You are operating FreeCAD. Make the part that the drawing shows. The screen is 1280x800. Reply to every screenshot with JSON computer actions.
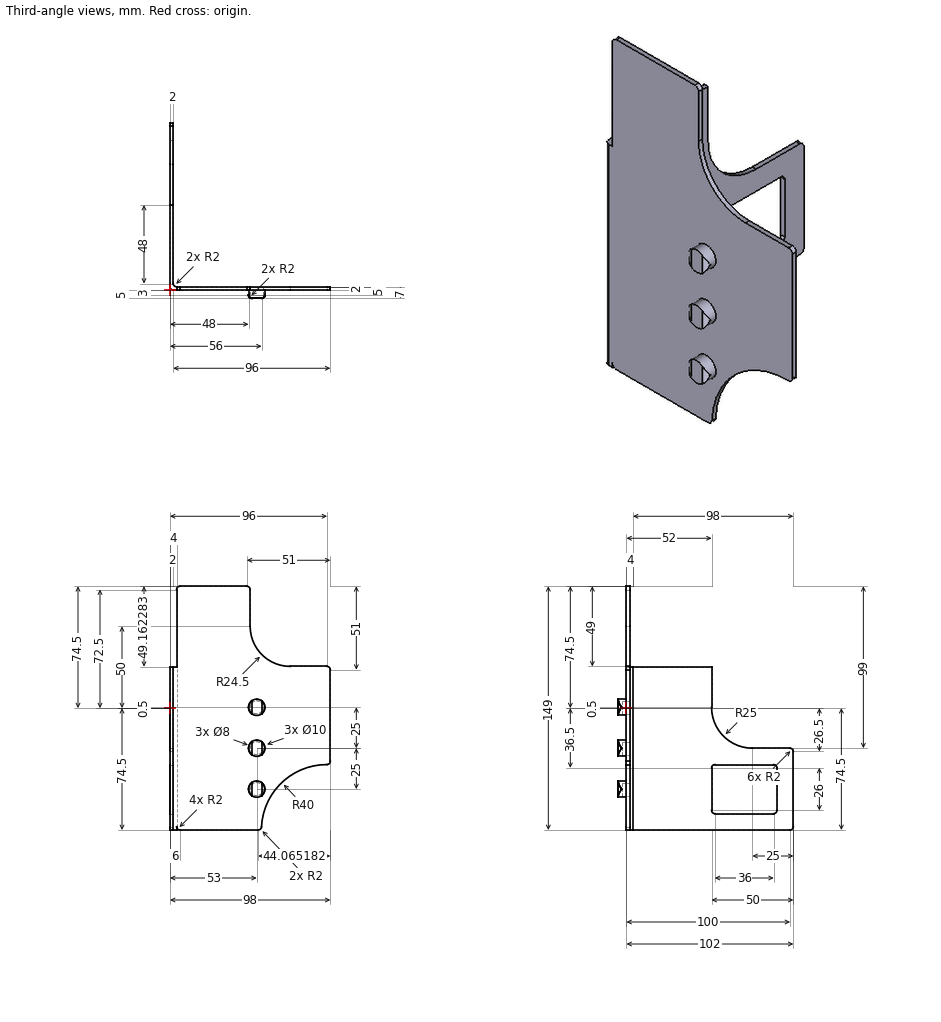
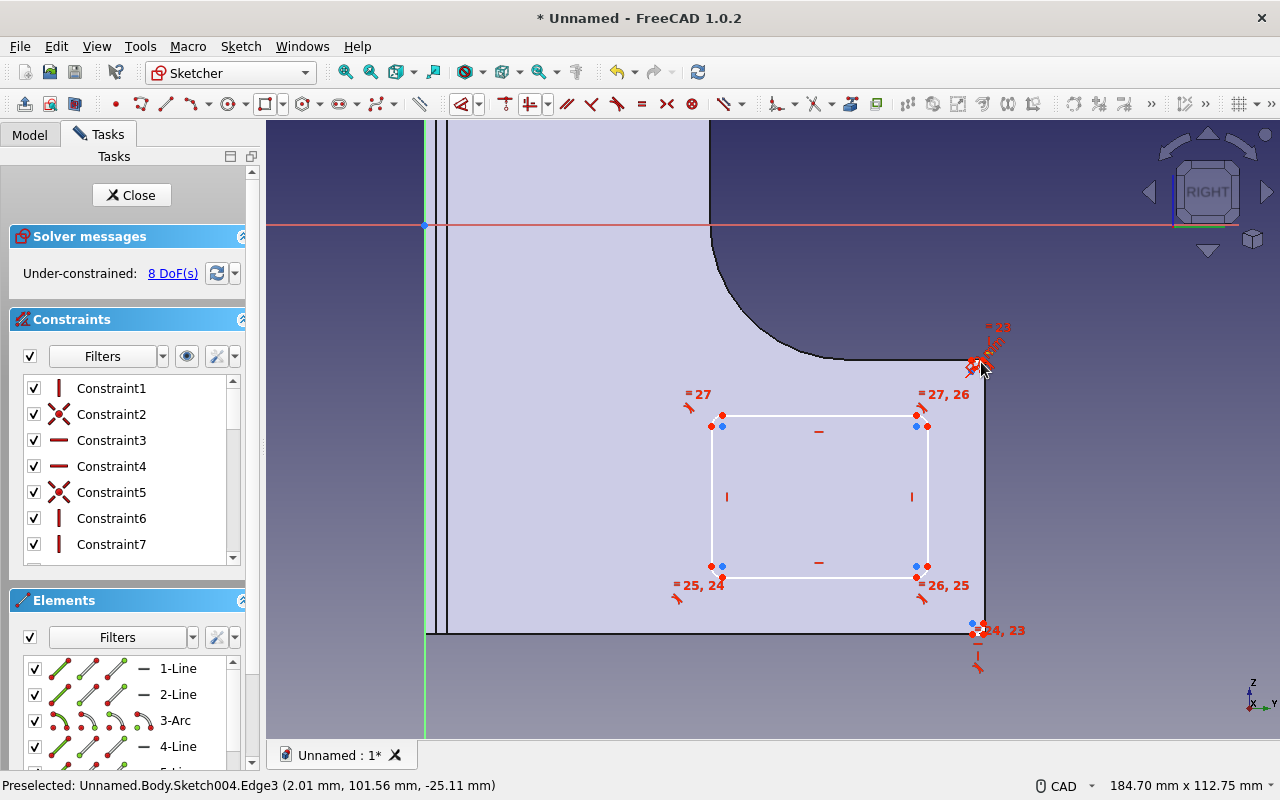
{"action": "left_click", "coordinate": [712, 469]}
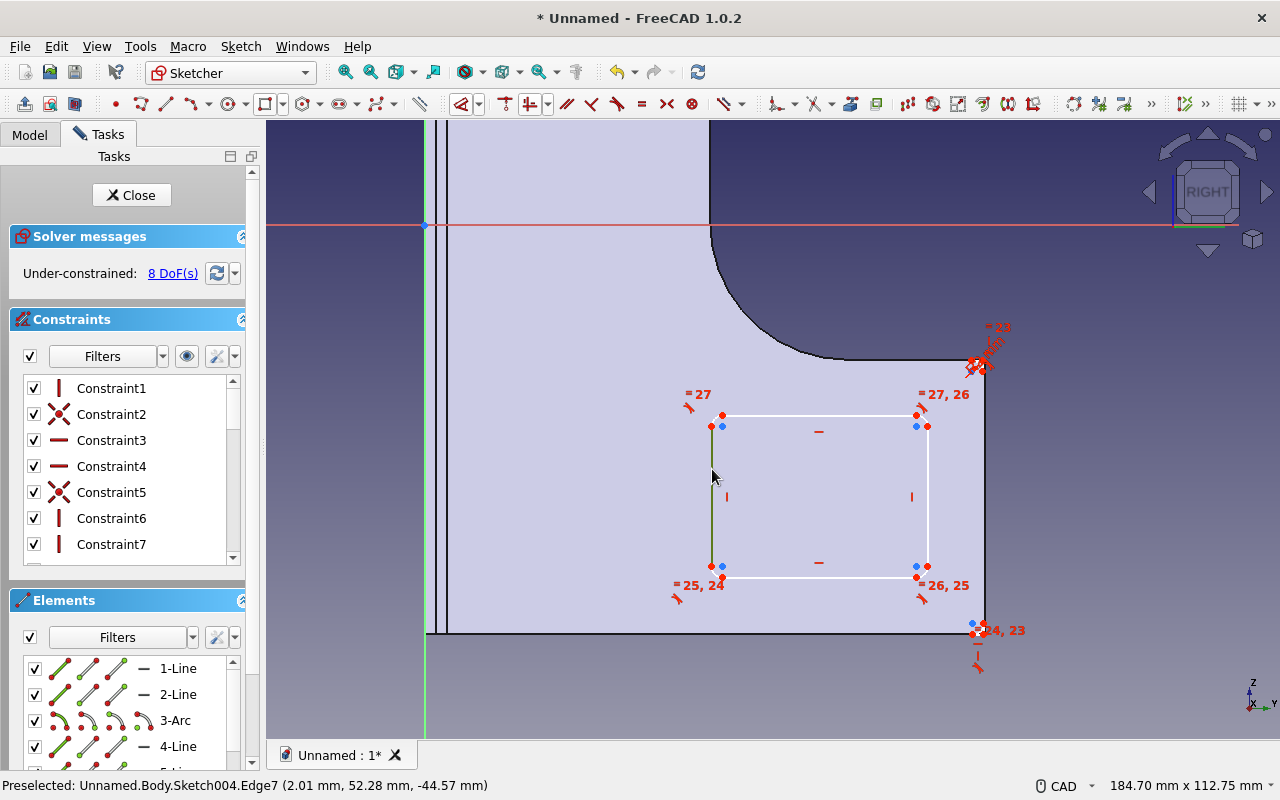
{"action": "key", "text": "i"}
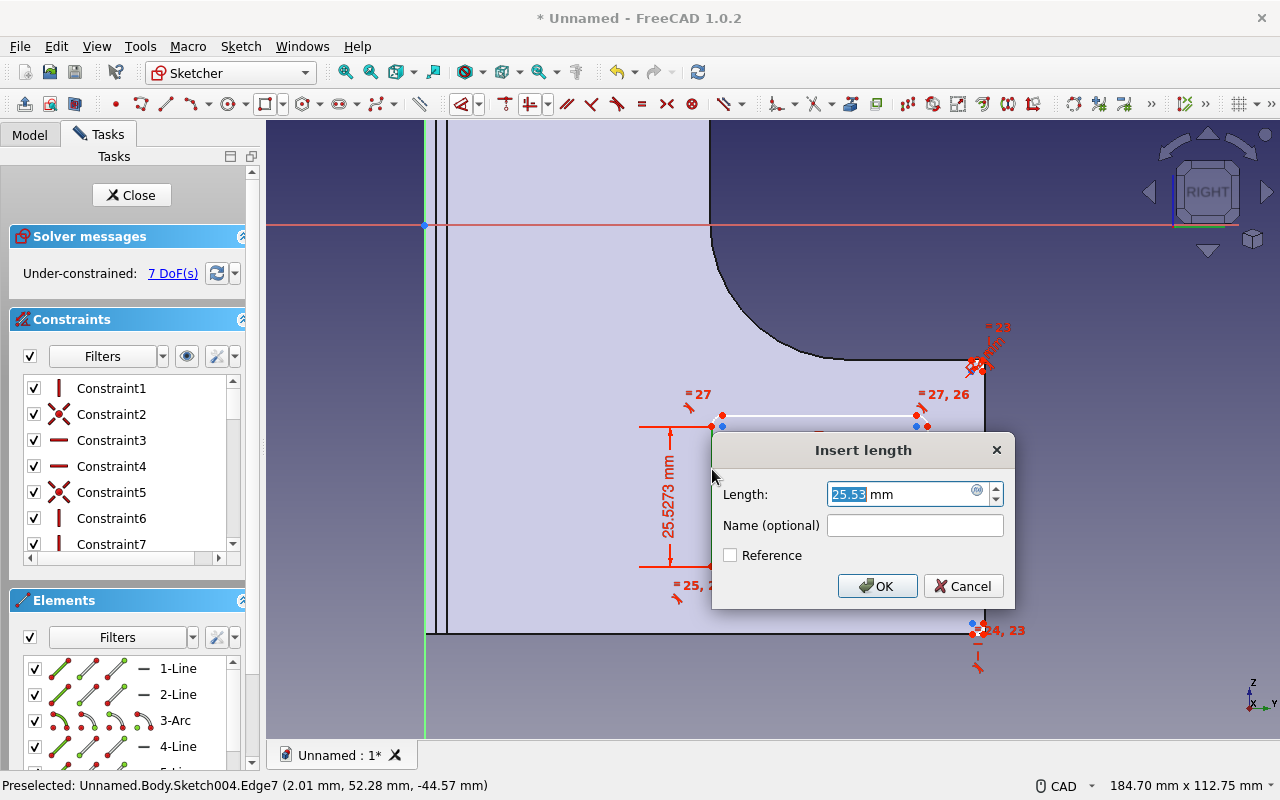
{"action": "type", "text": "26"}
{"action": "key", "text": "Return"}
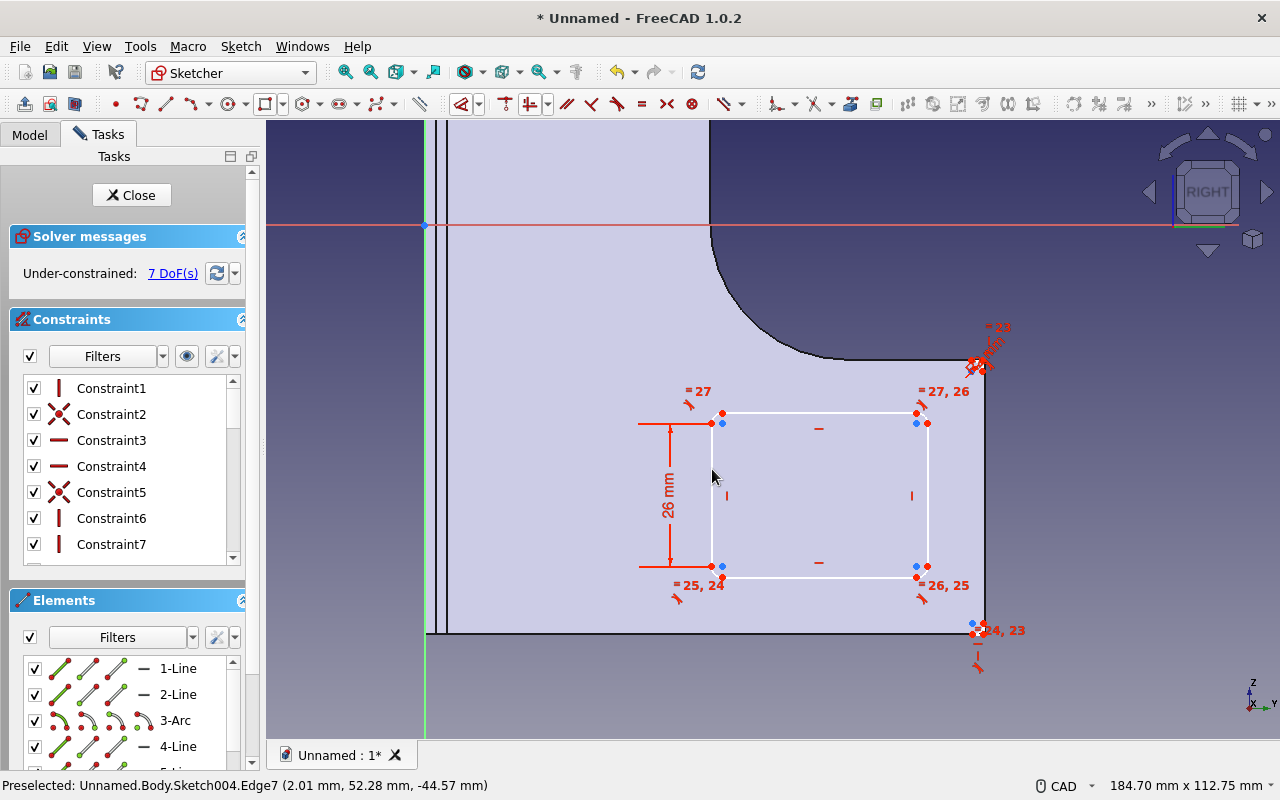
{"action": "left_click", "coordinate": [781, 578]}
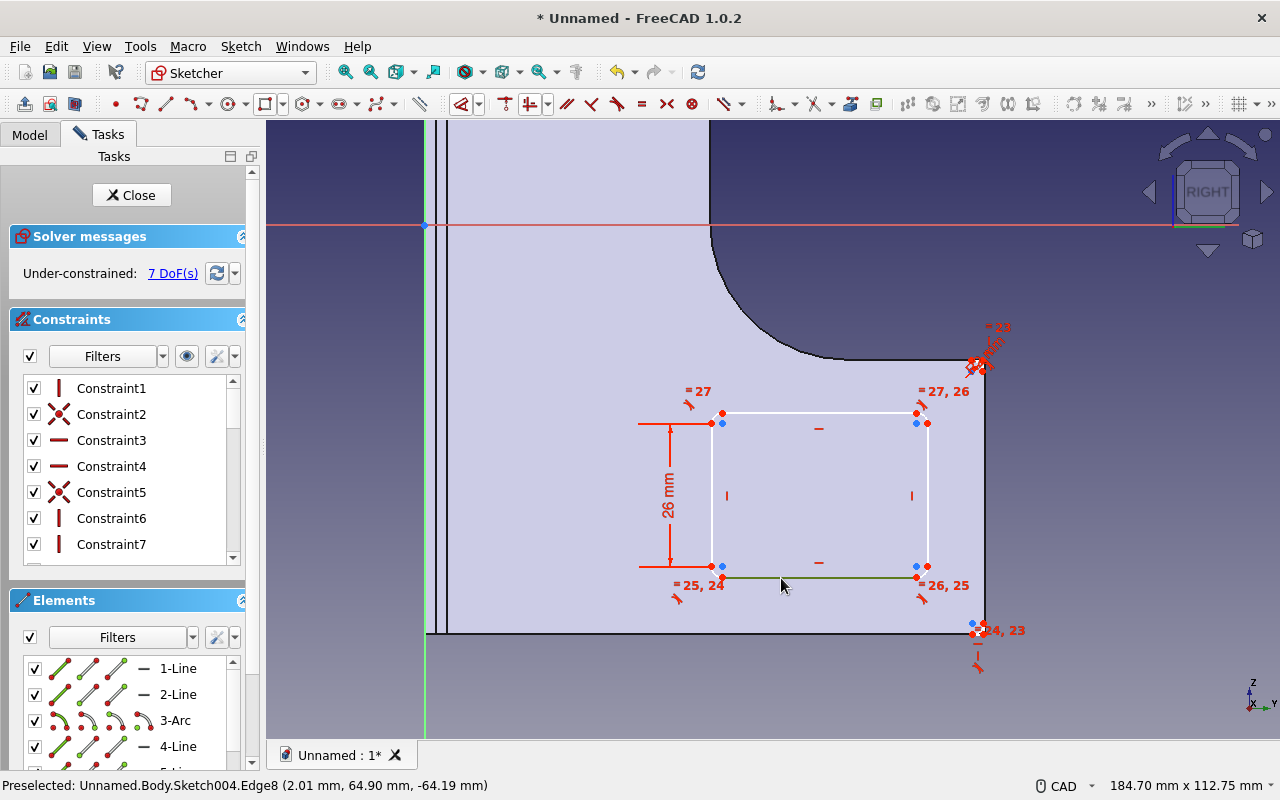
{"action": "key", "text": "l"}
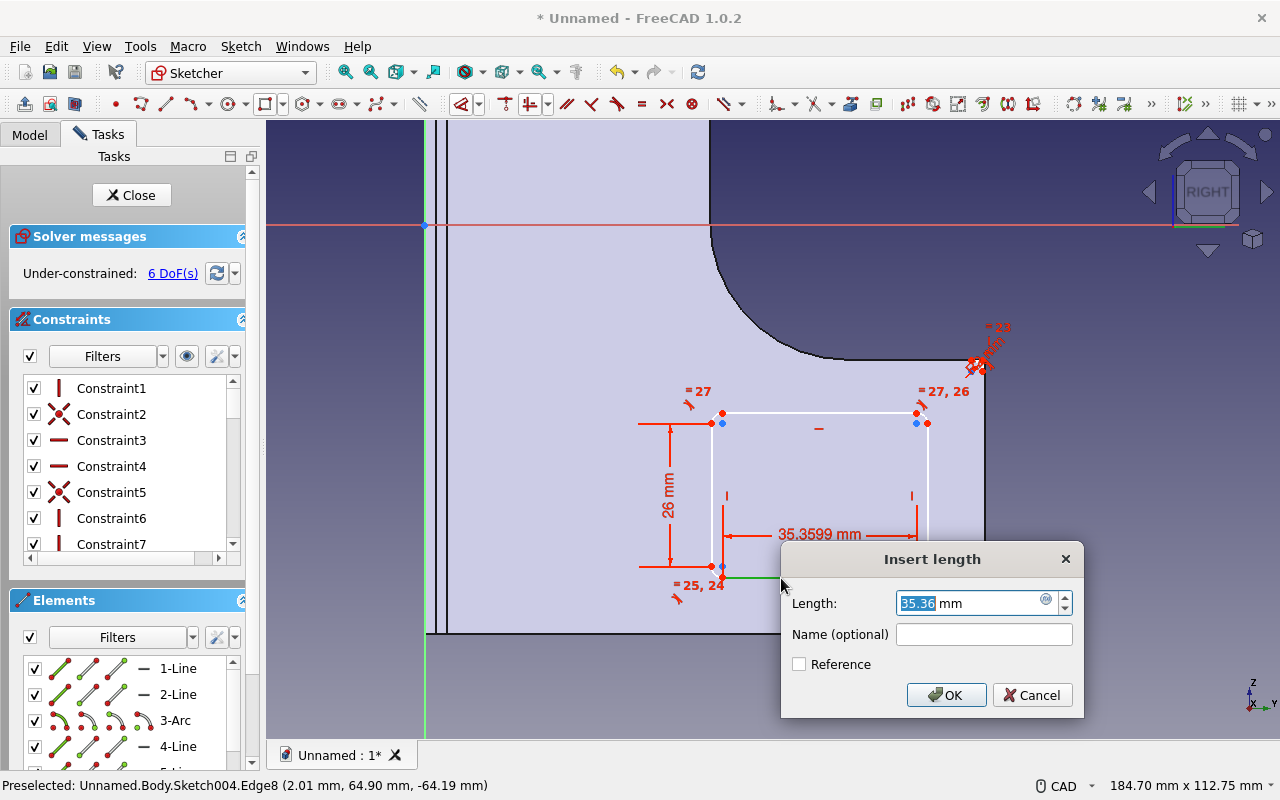
{"action": "type", "text": "36"}
{"action": "key", "text": "Return"}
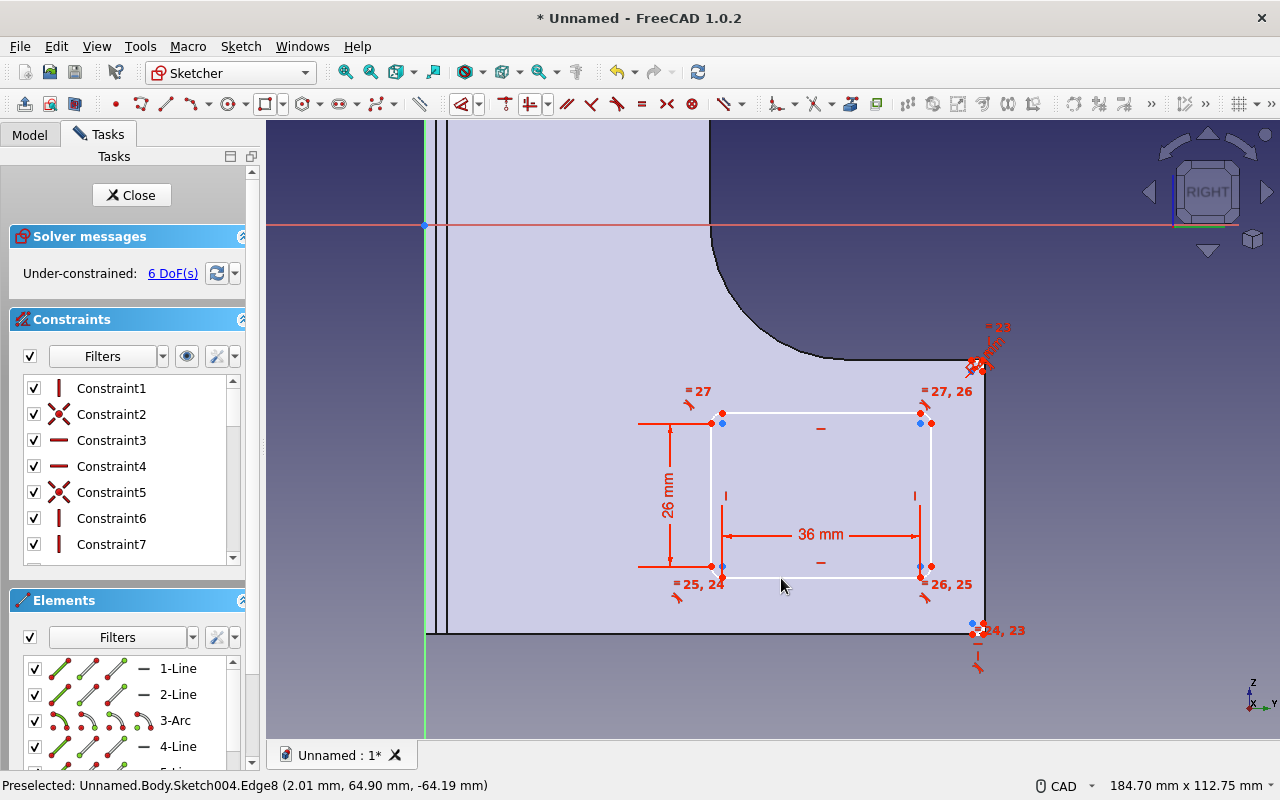
{"action": "left_click", "coordinate": [711, 424]}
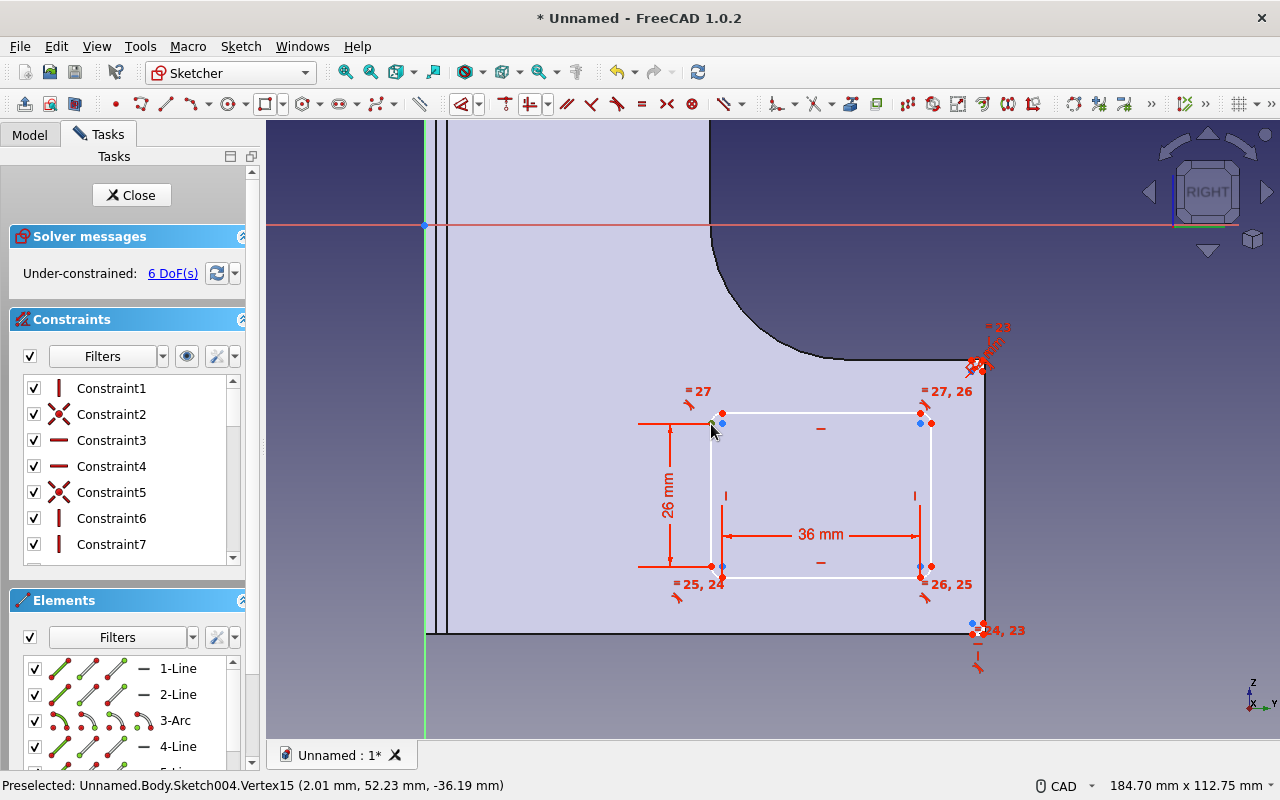
{"action": "key", "text": "l"}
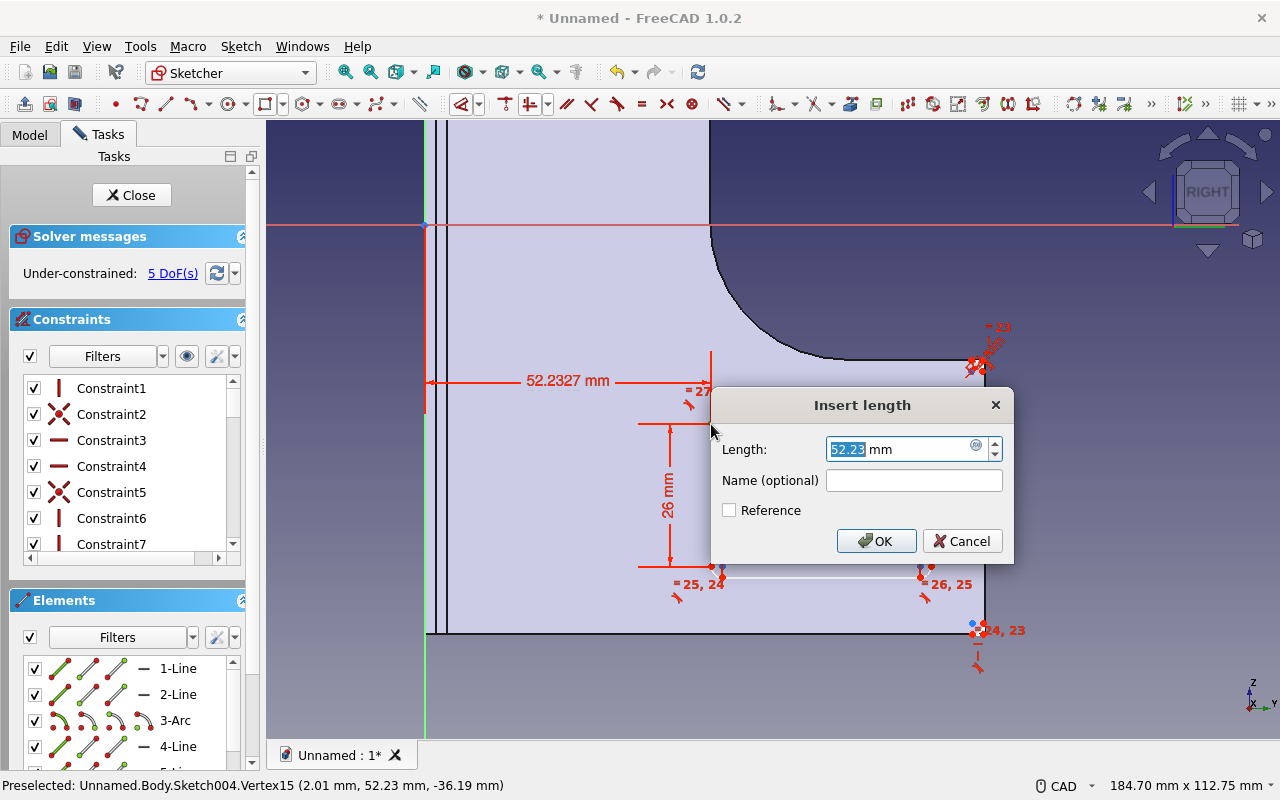
{"action": "type", "text": "52"}
{"action": "key", "text": "Return"}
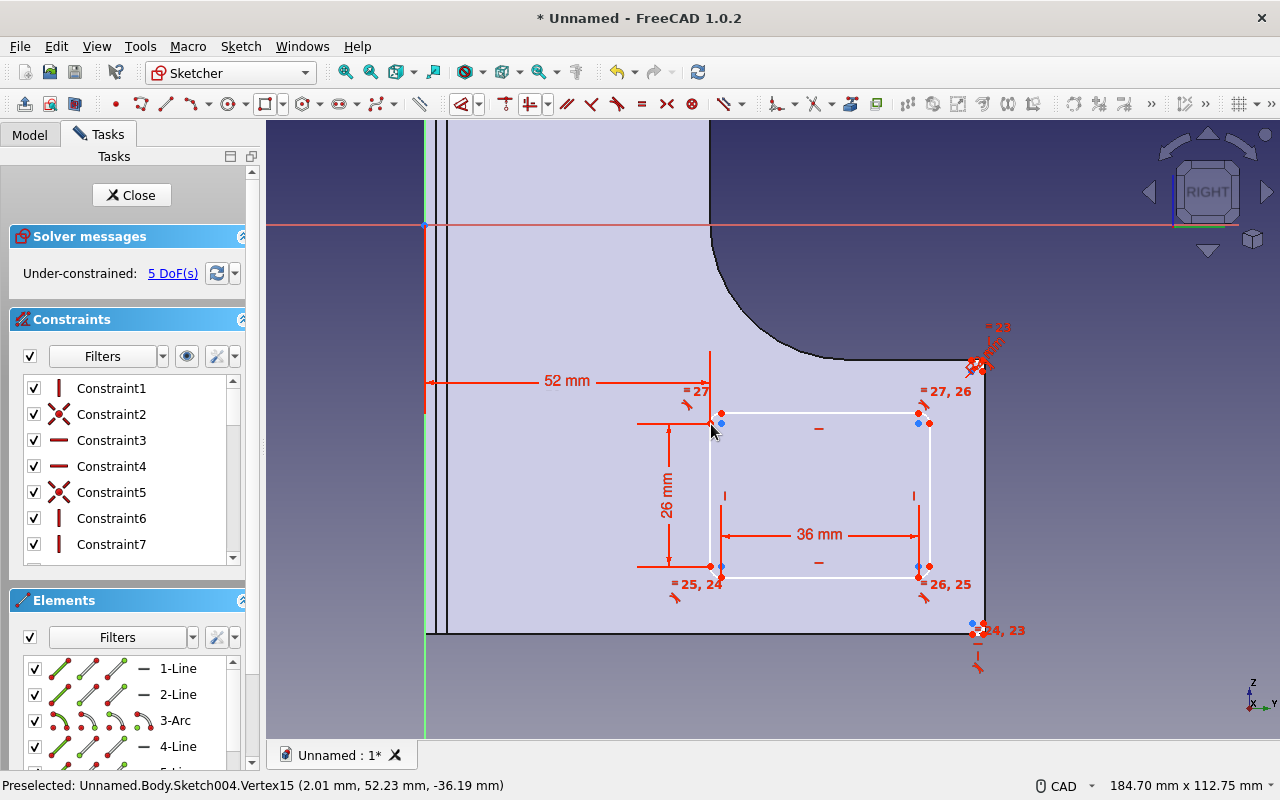
{"action": "left_click", "coordinate": [983, 372]}